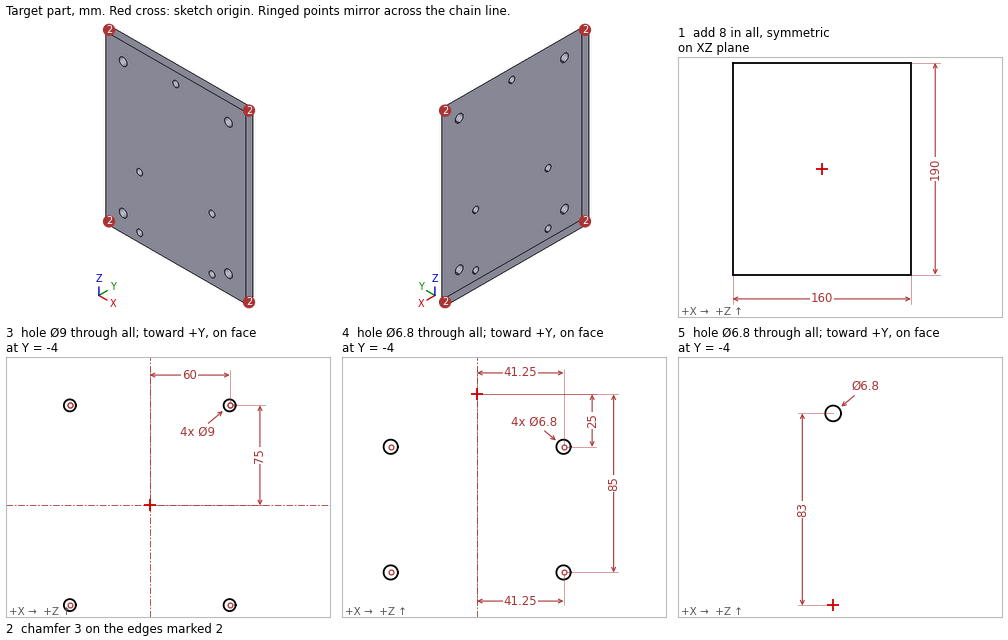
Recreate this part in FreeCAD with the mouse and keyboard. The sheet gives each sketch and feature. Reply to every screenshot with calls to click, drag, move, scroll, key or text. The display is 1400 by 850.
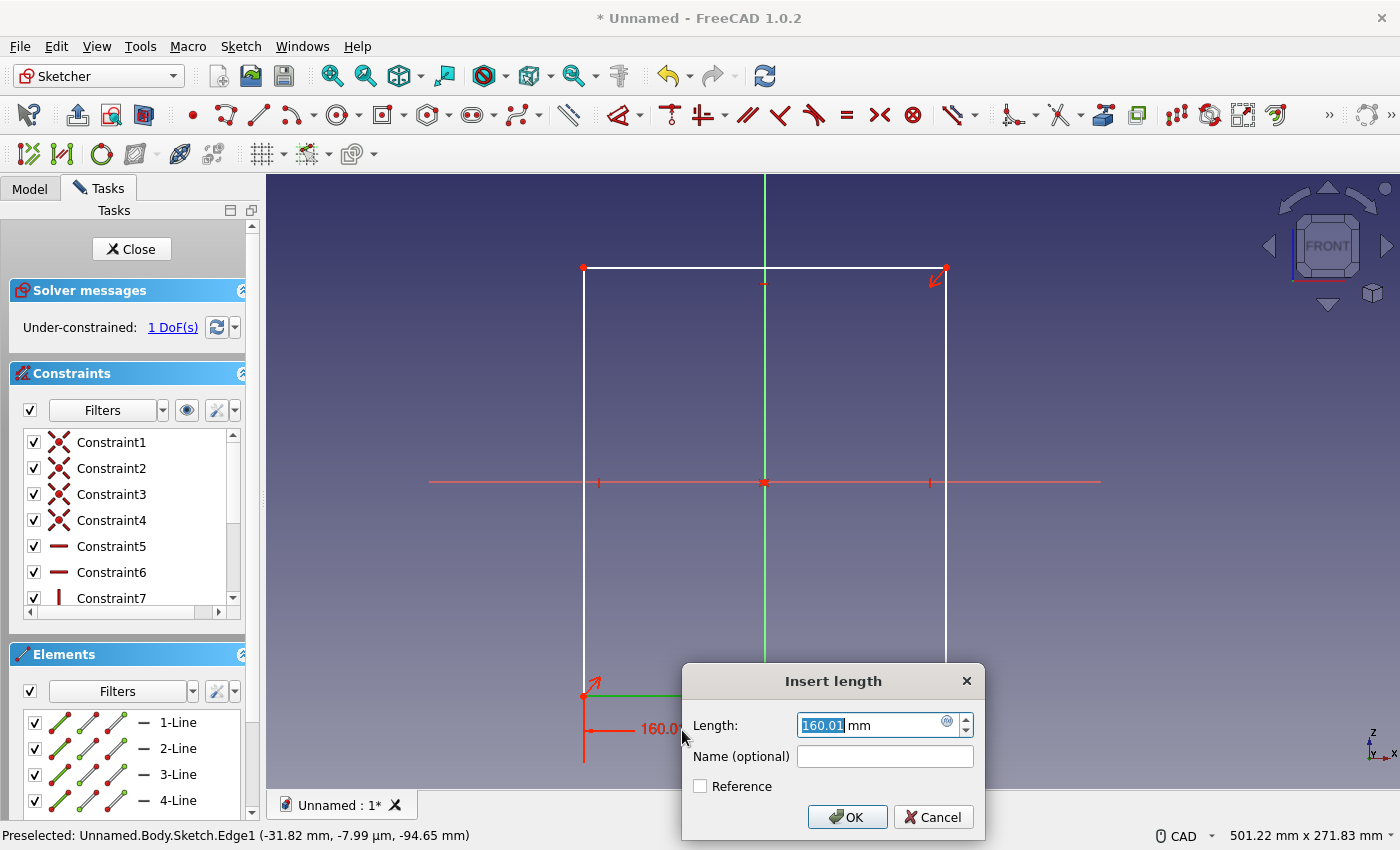
text(160)
key(Return)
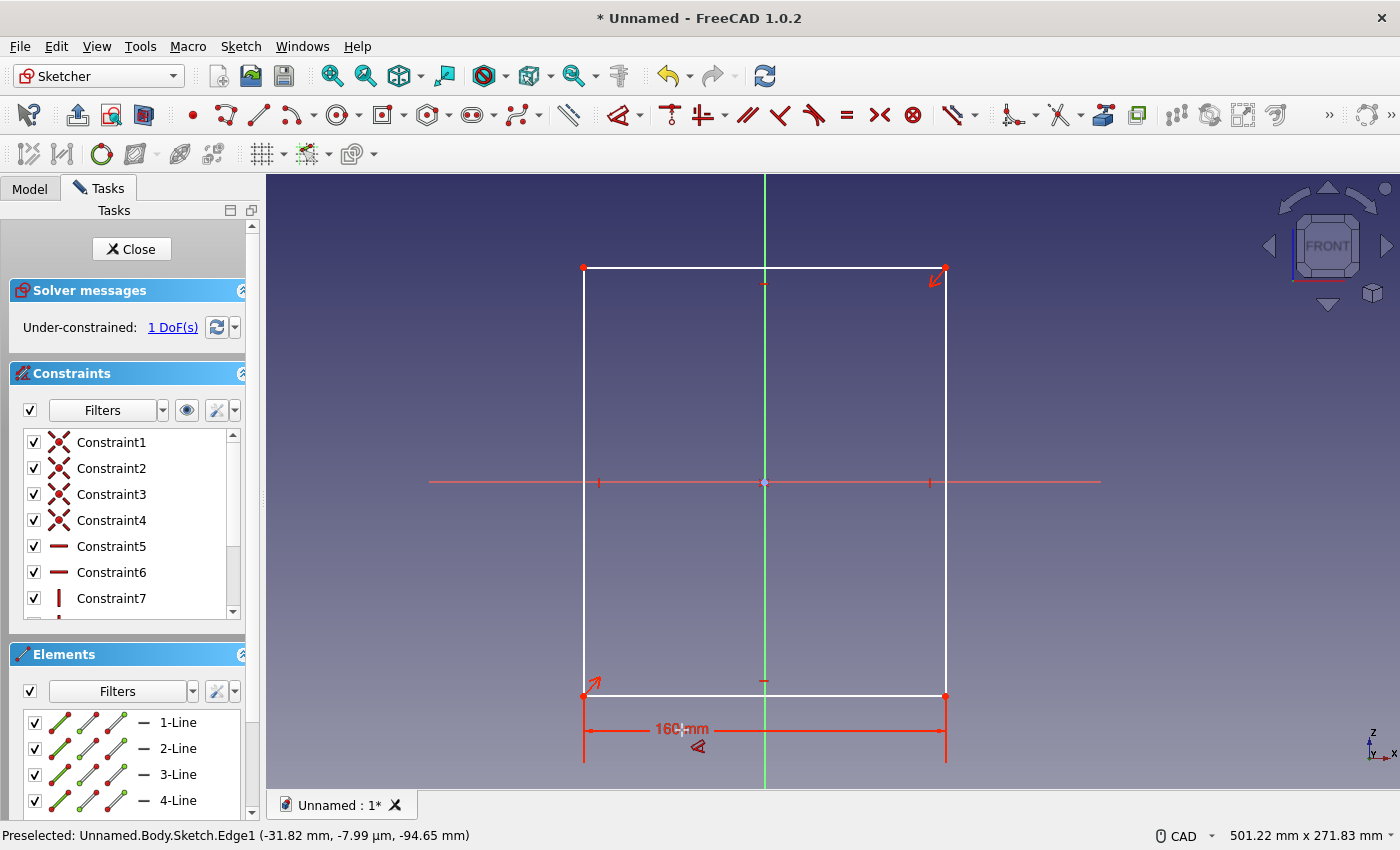
click(946, 568)
click(980, 384)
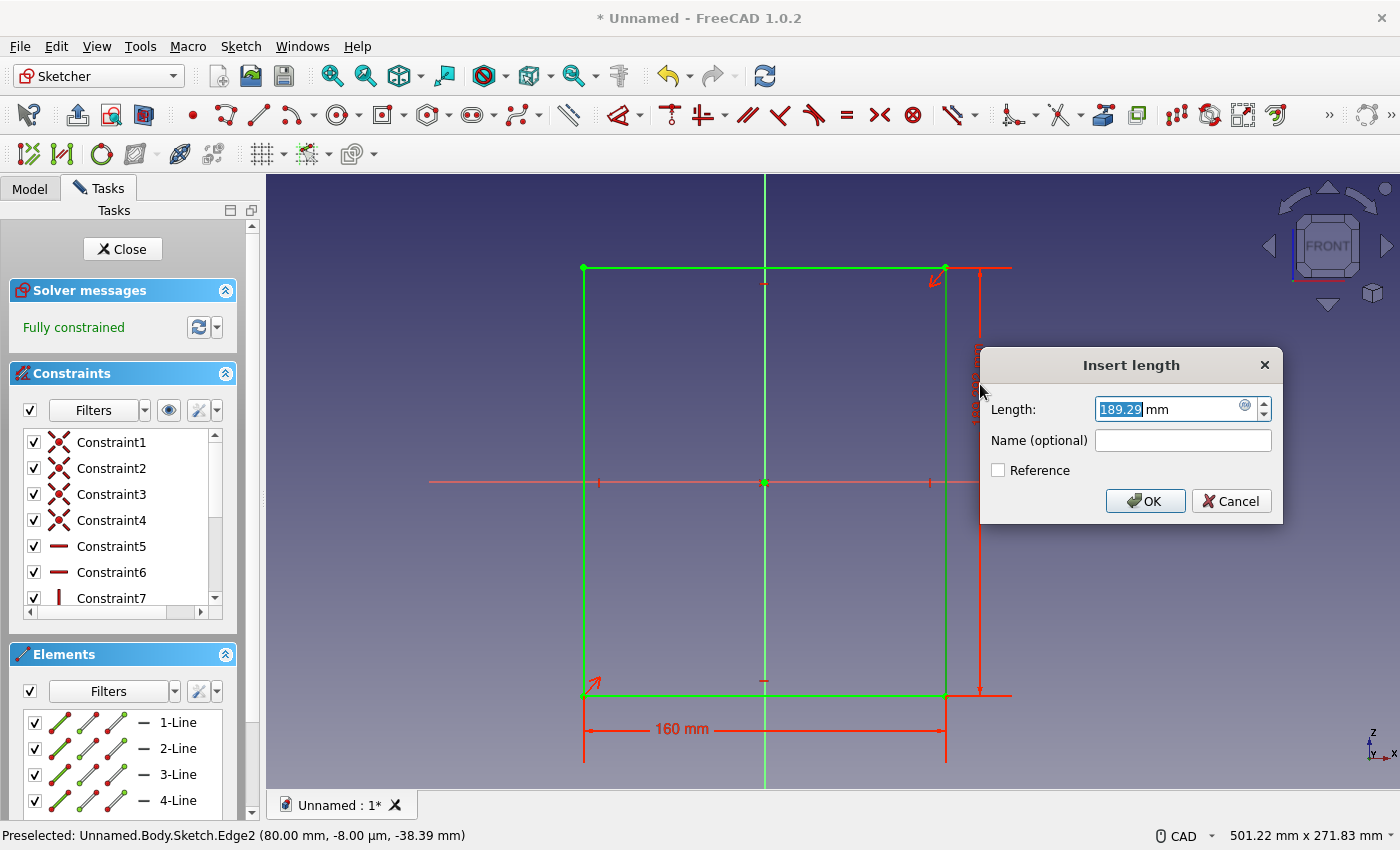
text(190)
key(Return)
key(Escape)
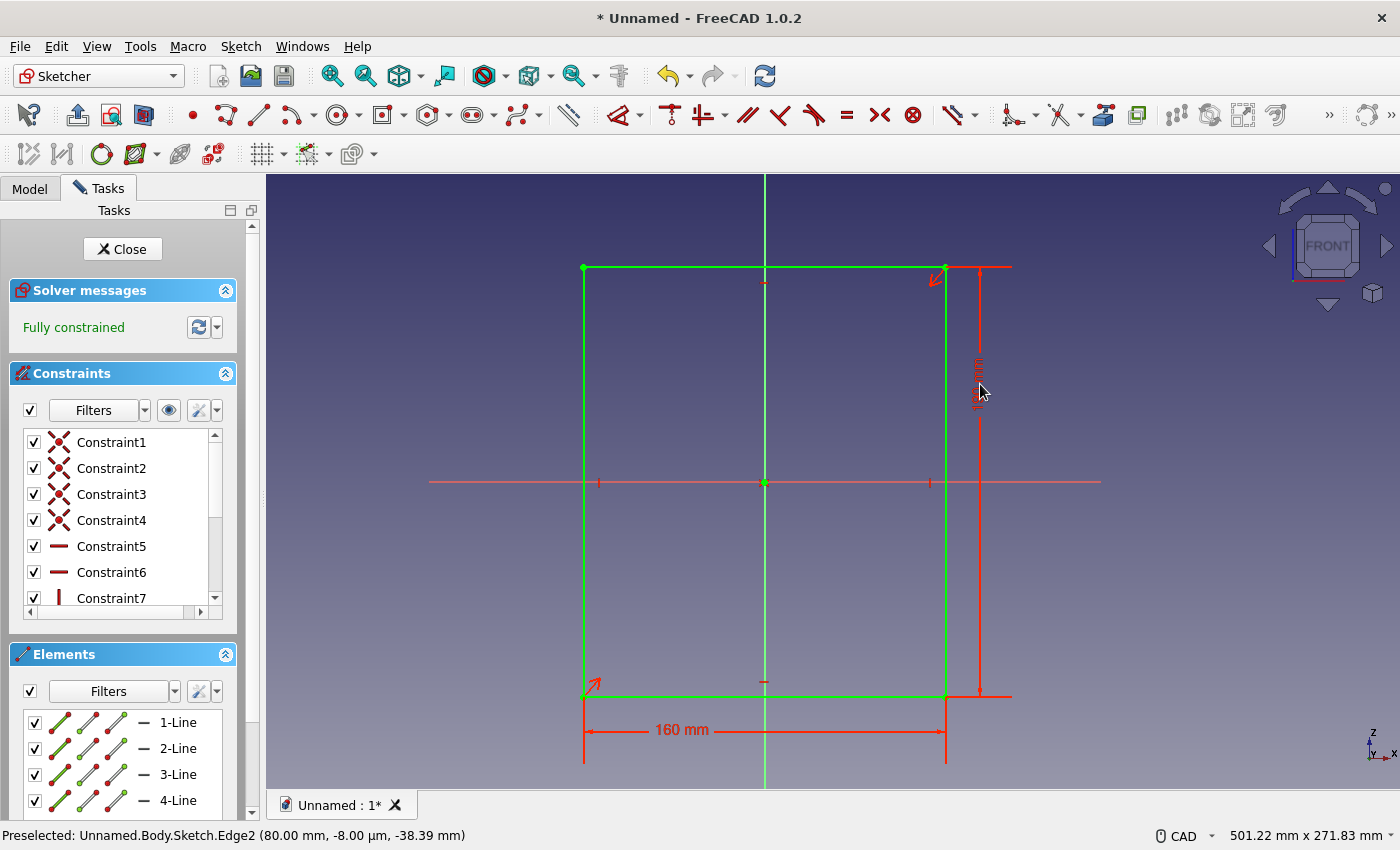
click(123, 249)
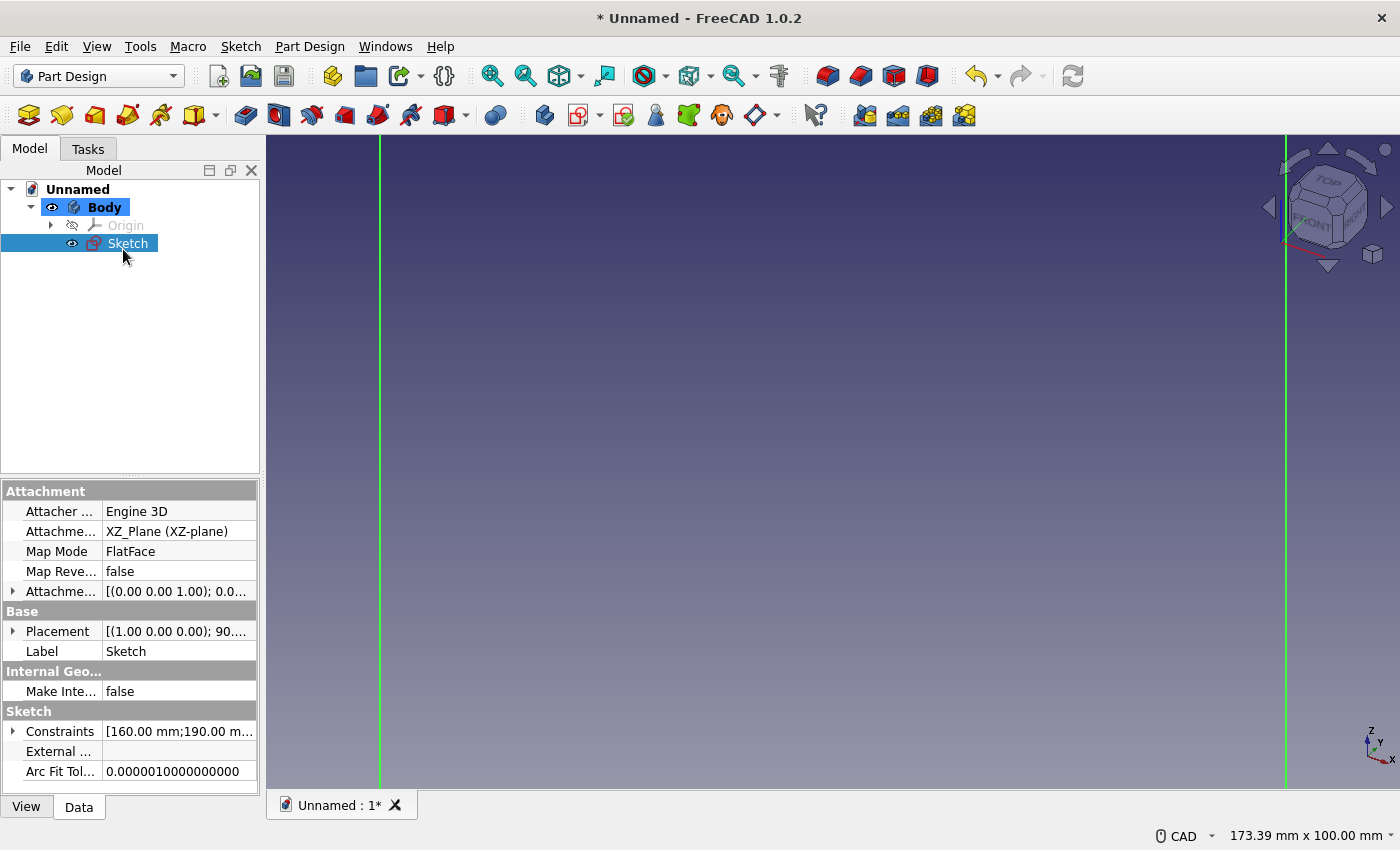
click(29, 116)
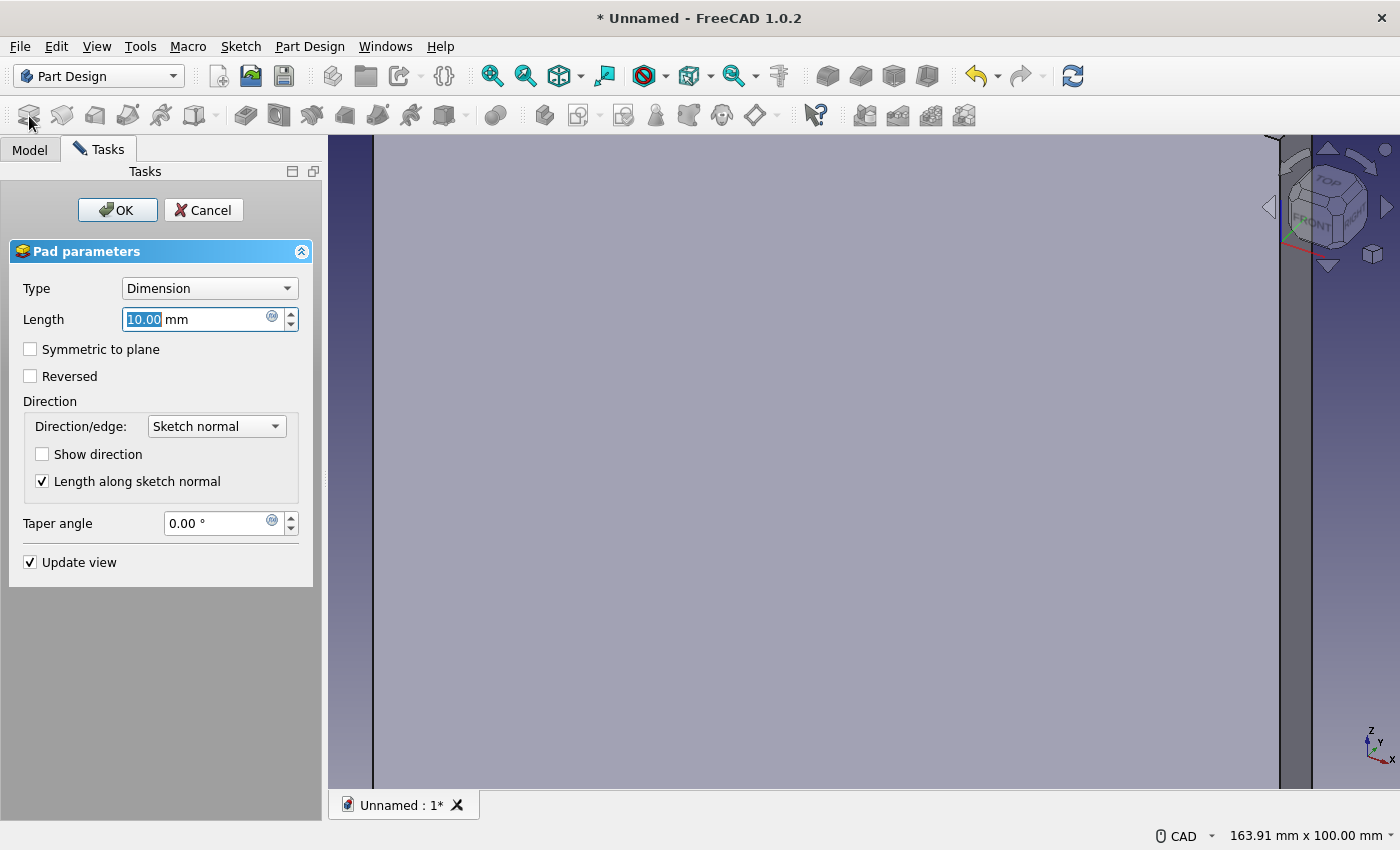
text(8)
key(Tab)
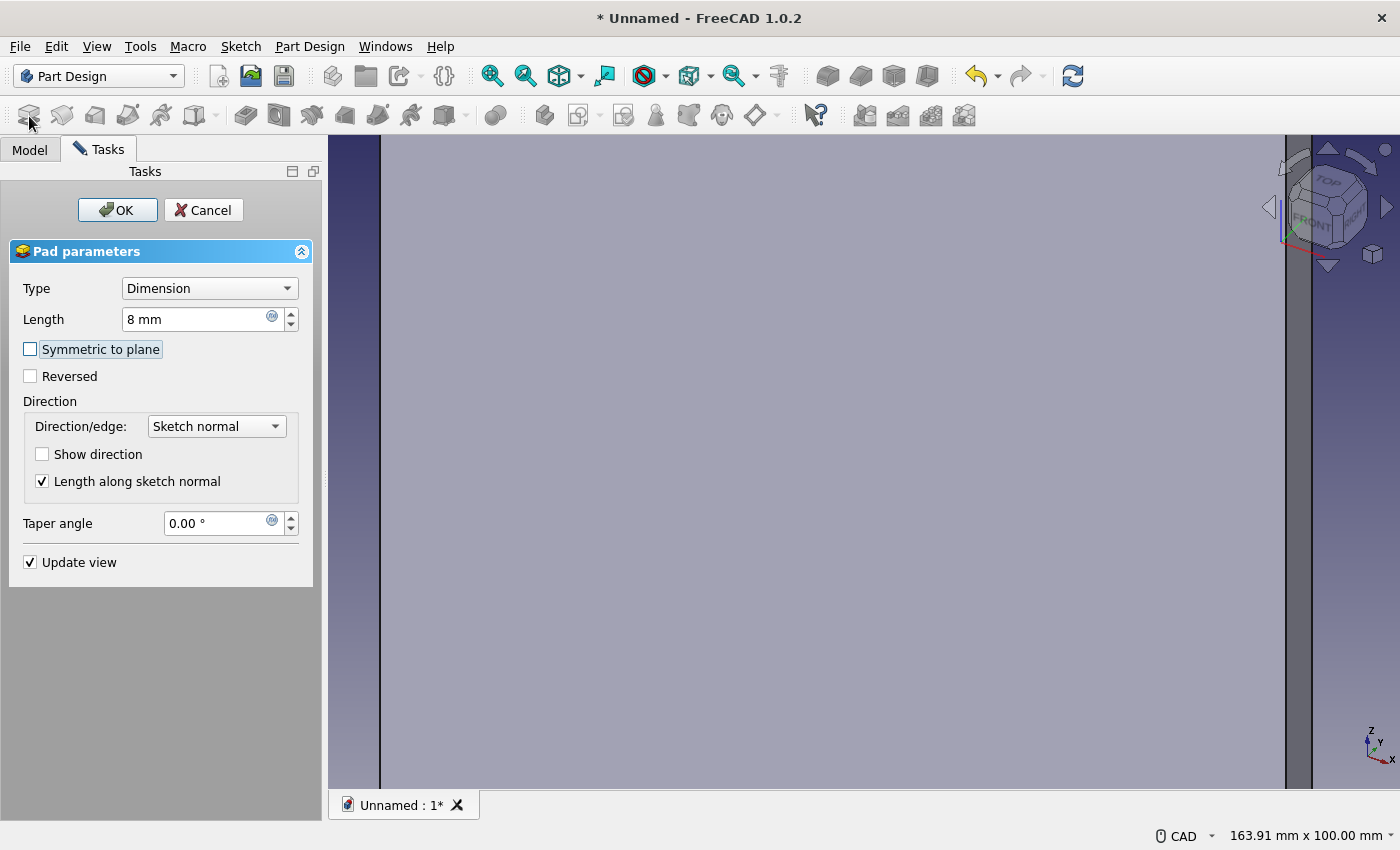
click(31, 349)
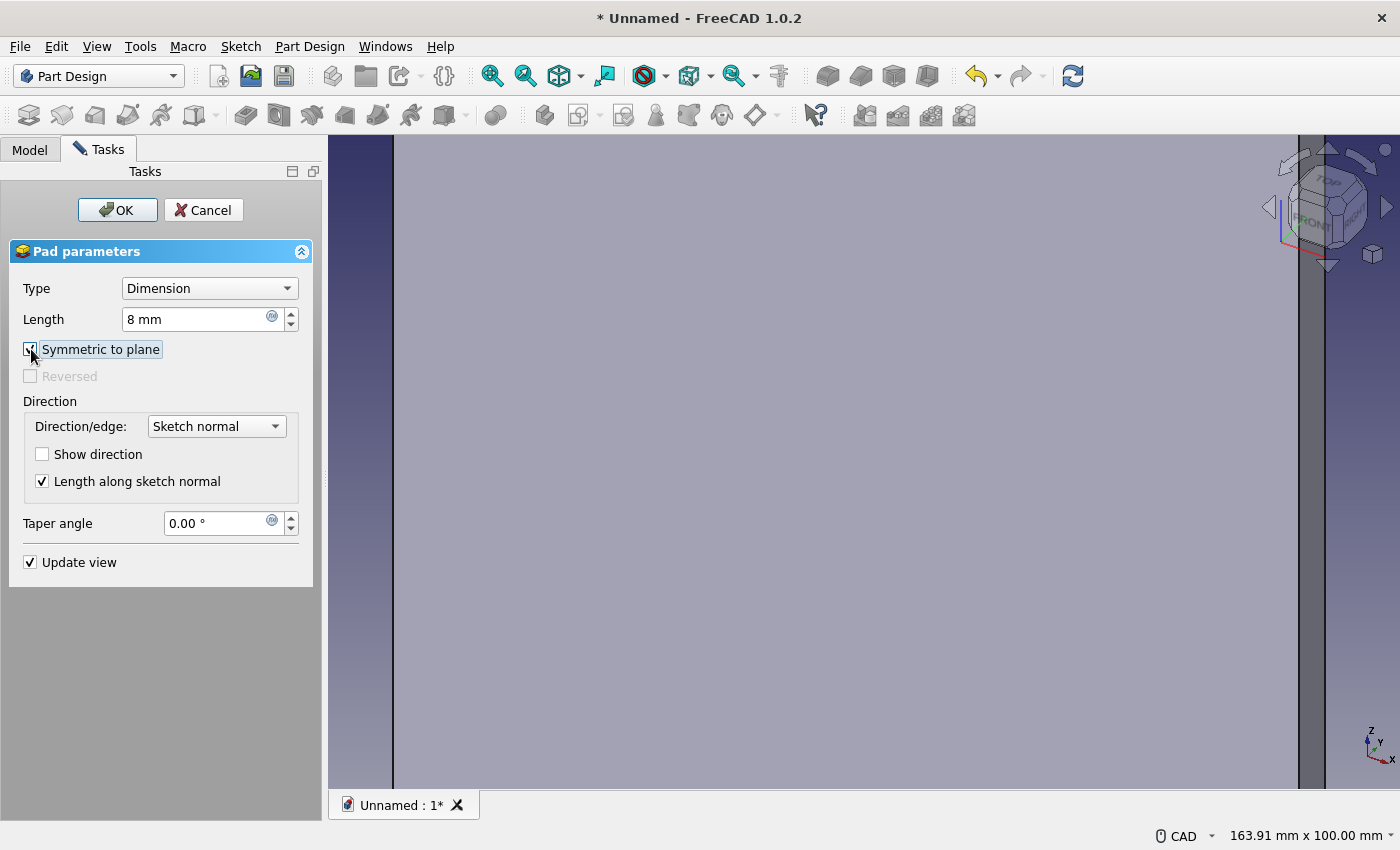
click(118, 210)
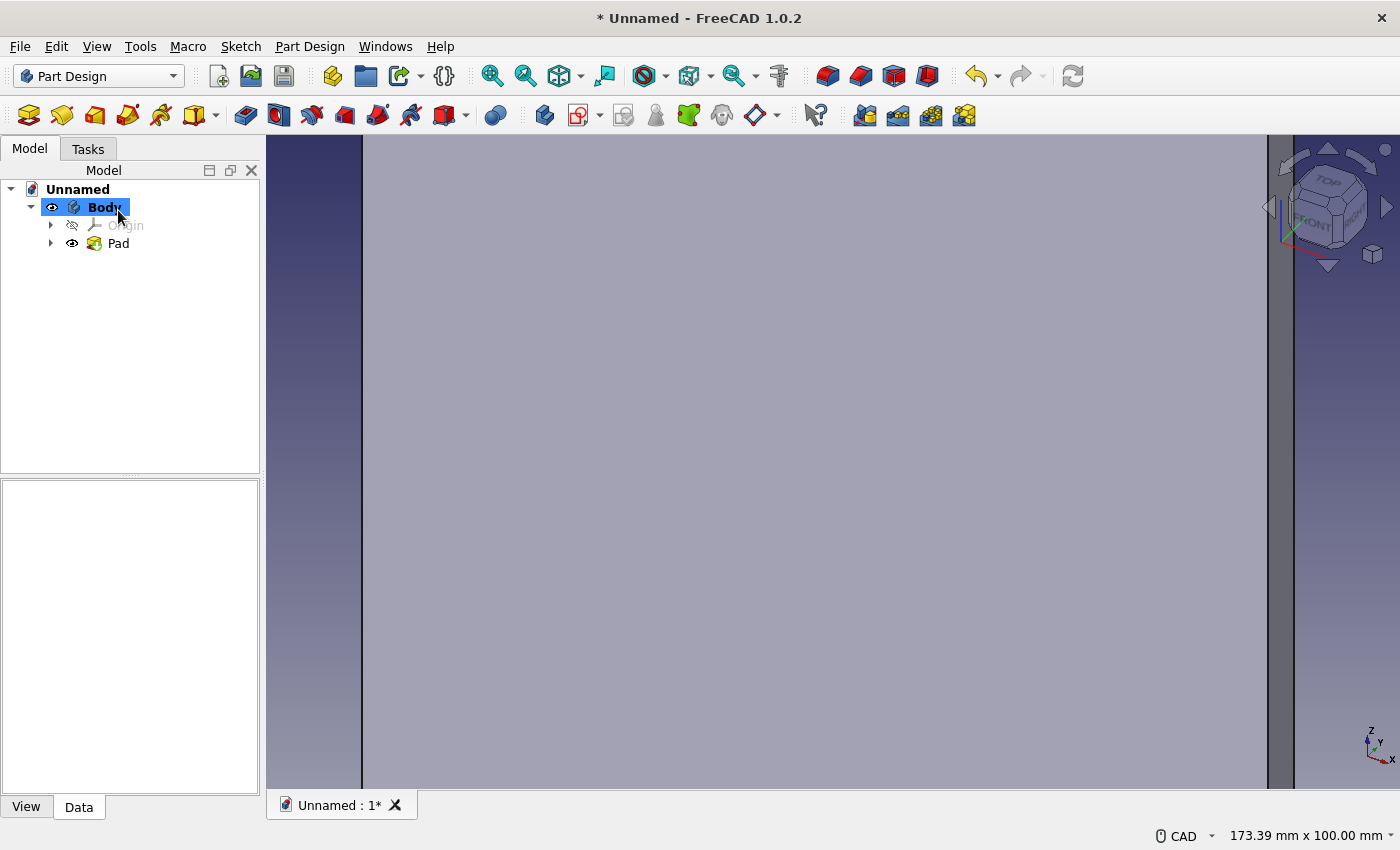
click(493, 76)